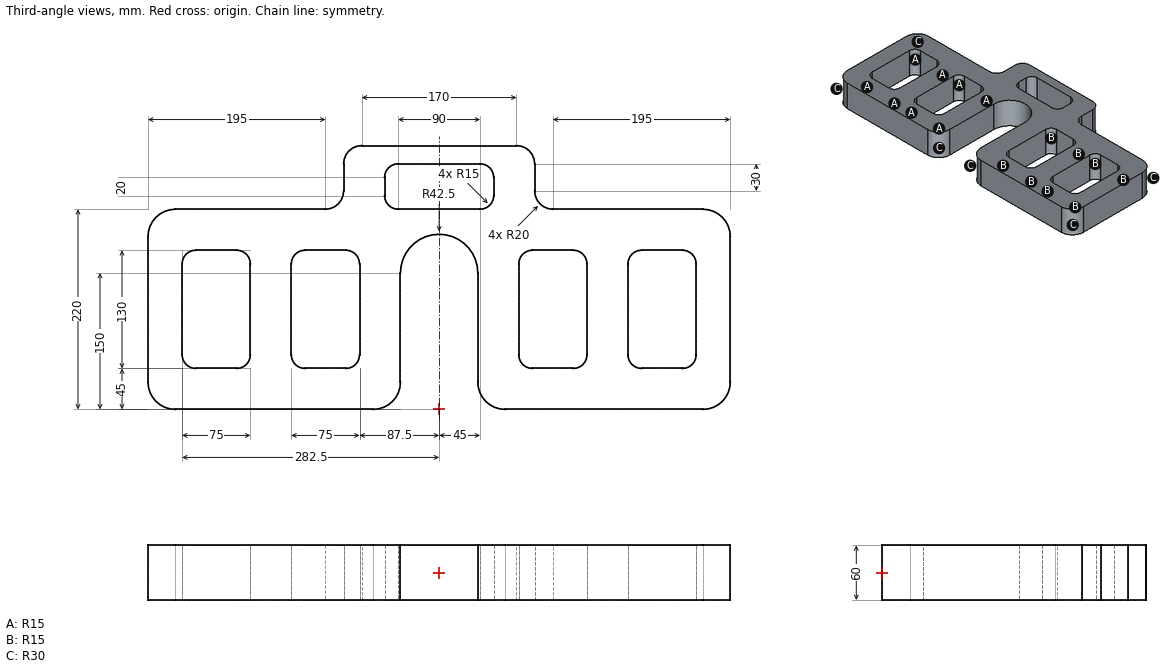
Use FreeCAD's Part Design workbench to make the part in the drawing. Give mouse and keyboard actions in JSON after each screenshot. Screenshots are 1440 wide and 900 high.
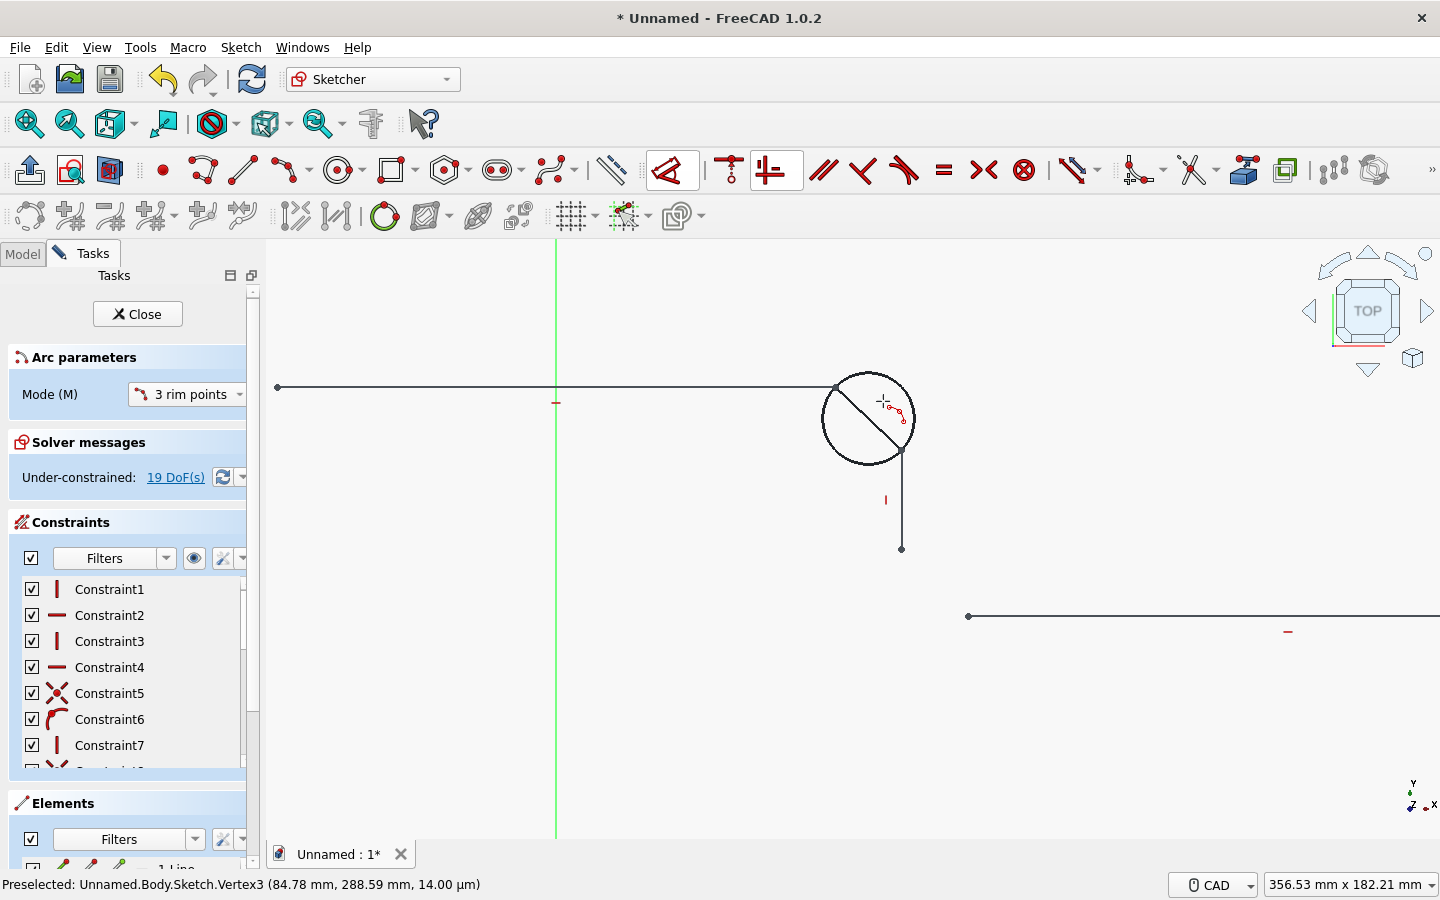
{"action": "left_click", "coordinate": [883, 402]}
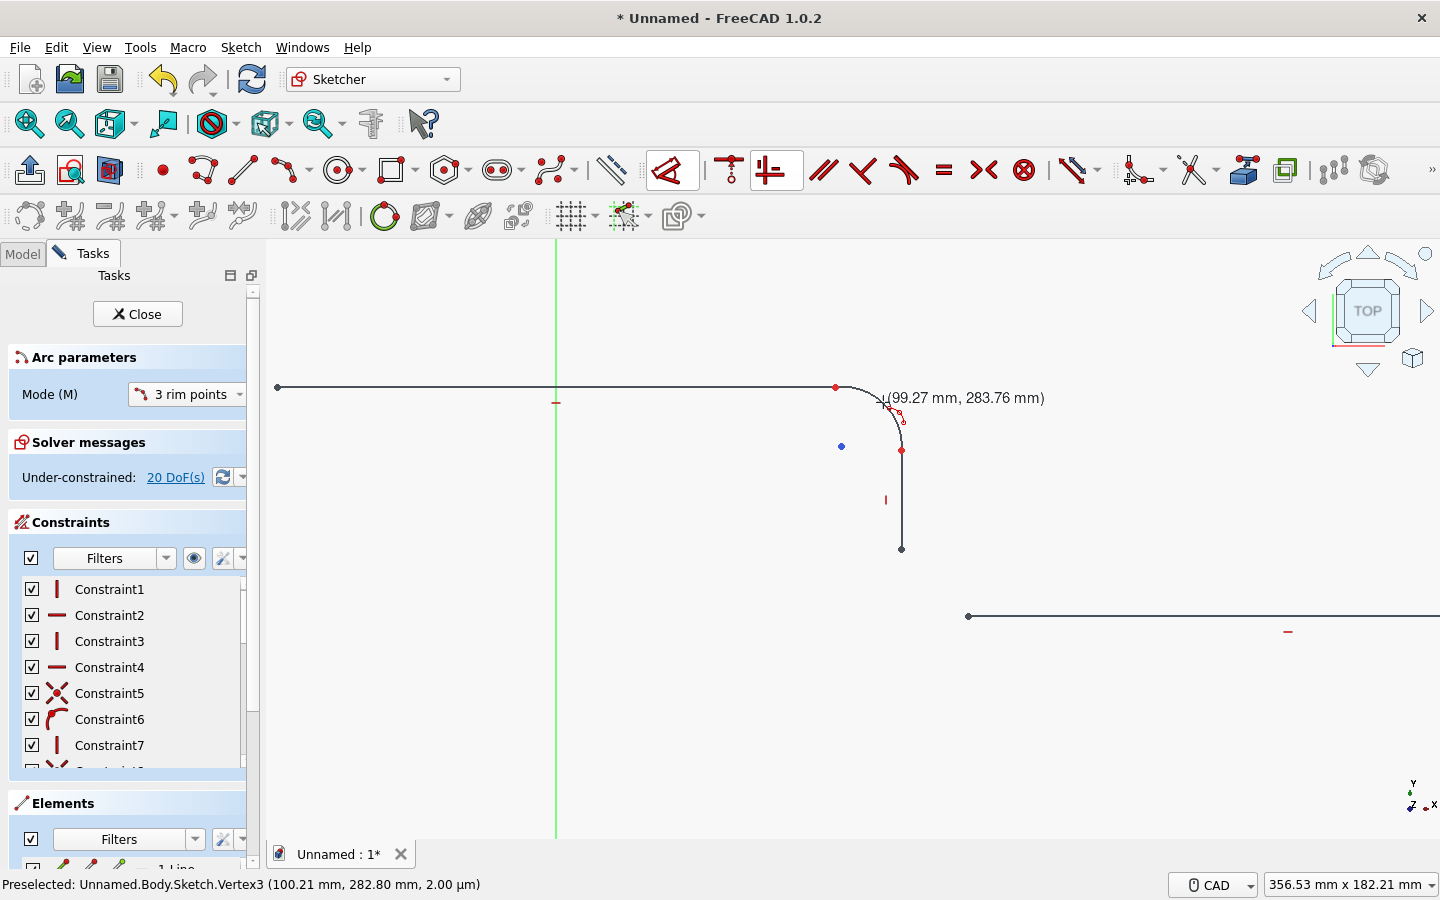
{"action": "scroll", "coordinate": [883, 401], "scroll_direction": "down", "scroll_amount": 6}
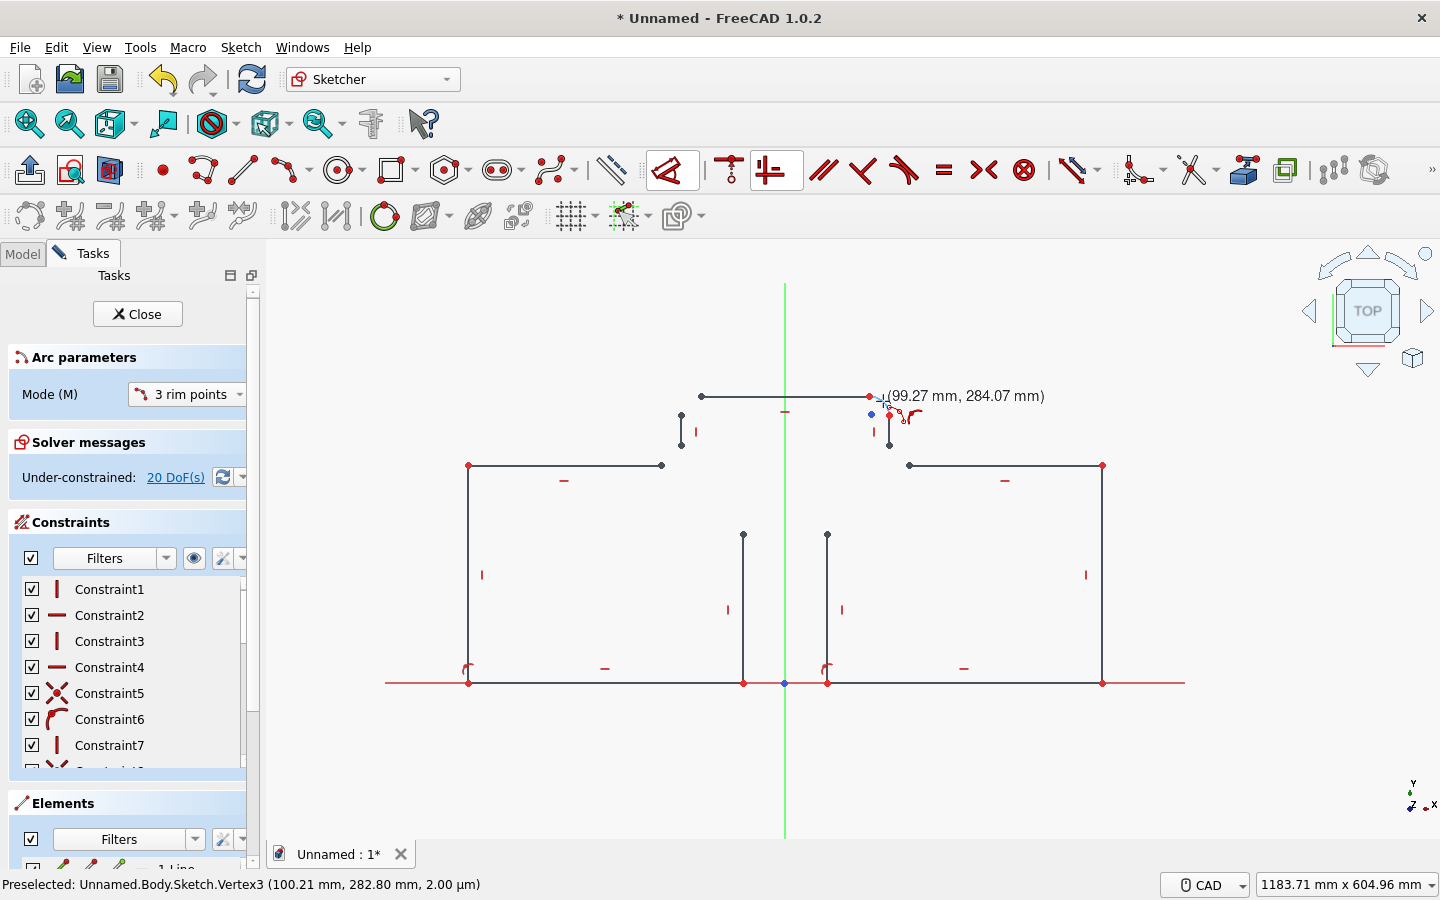
{"action": "left_click", "coordinate": [701, 397]}
{"action": "left_click", "coordinate": [681, 416]}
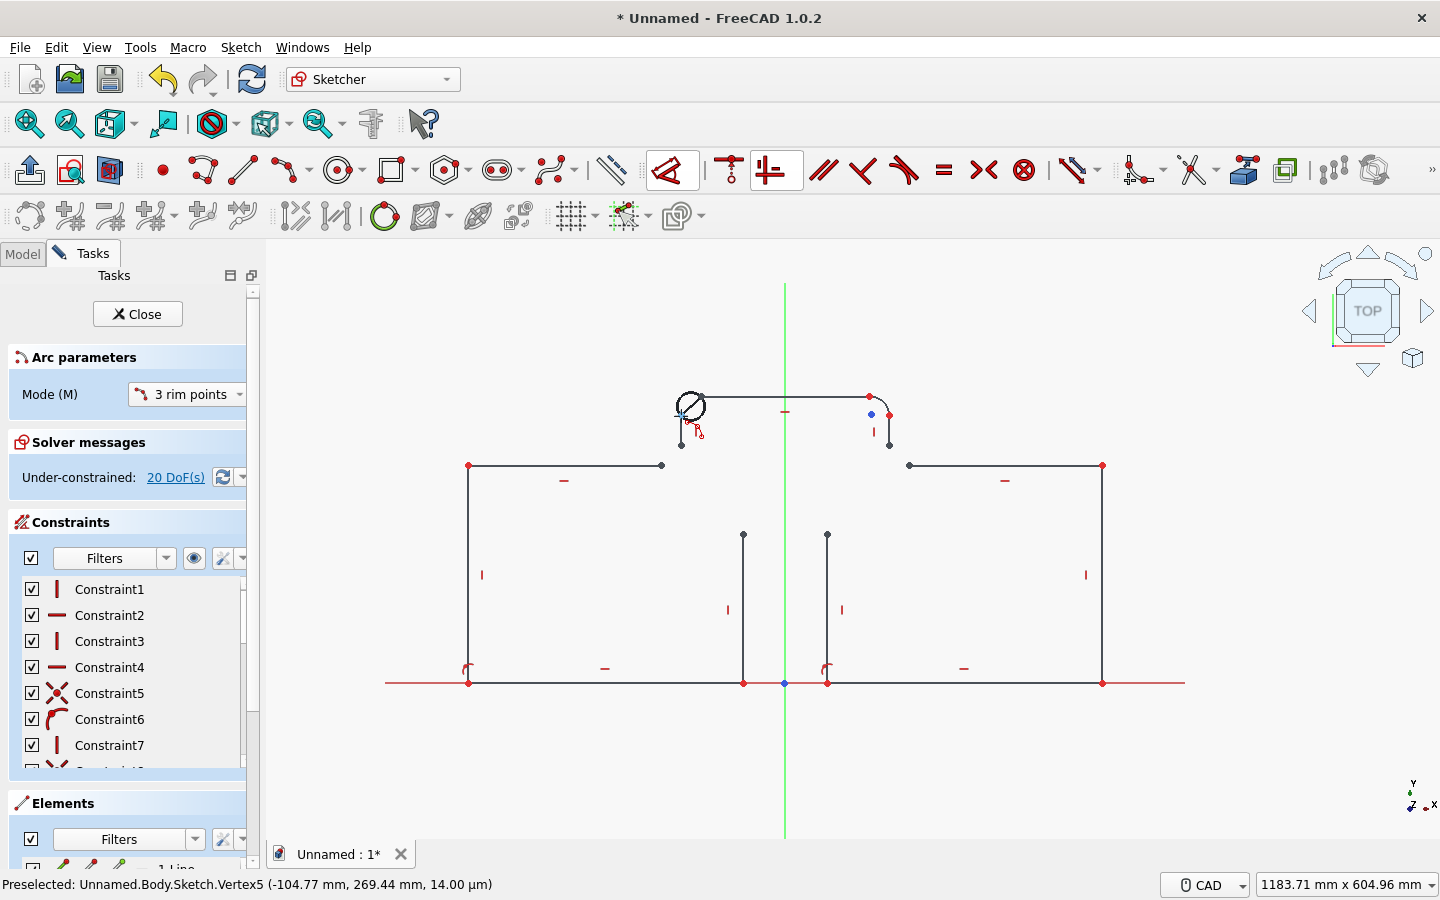
{"action": "scroll", "coordinate": [687, 401], "scroll_direction": "up", "scroll_amount": 6}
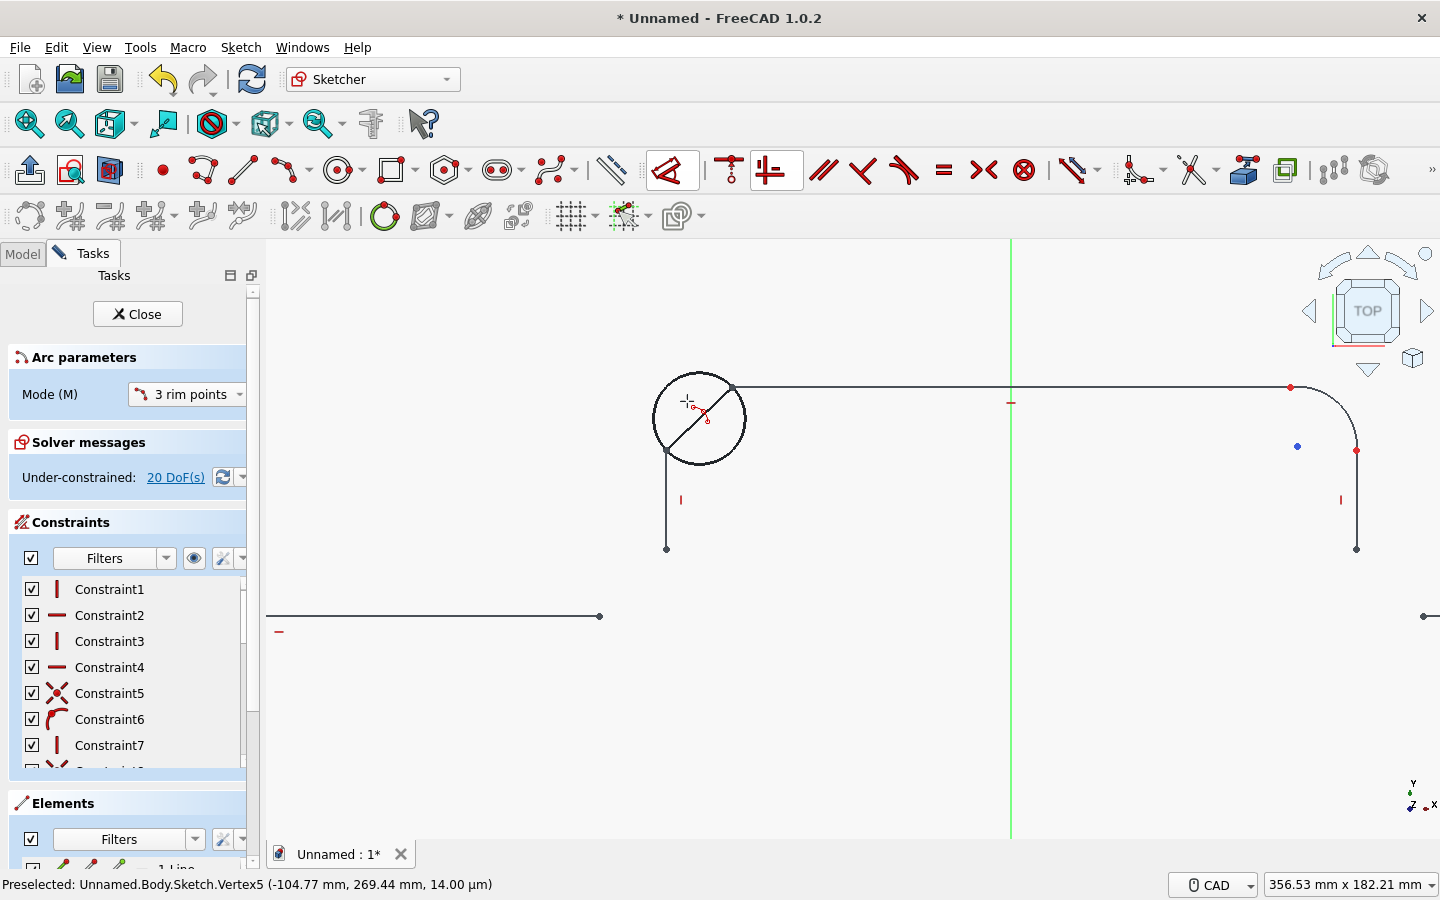
{"action": "left_click", "coordinate": [685, 402]}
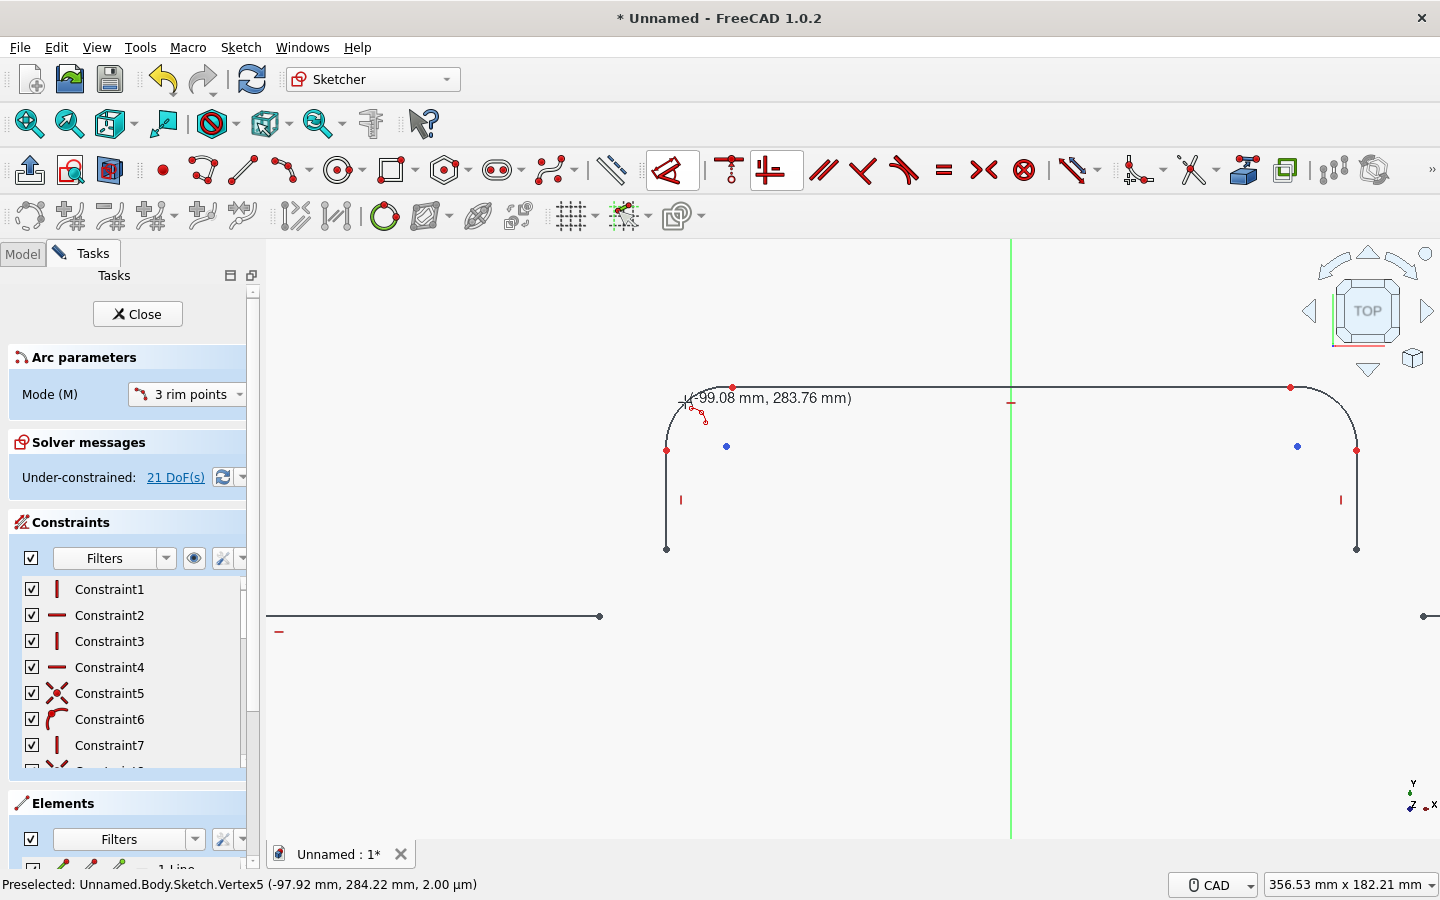
{"action": "left_click", "coordinate": [666, 550]}
{"action": "left_click", "coordinate": [600, 616]}
{"action": "left_click", "coordinate": [646, 594]}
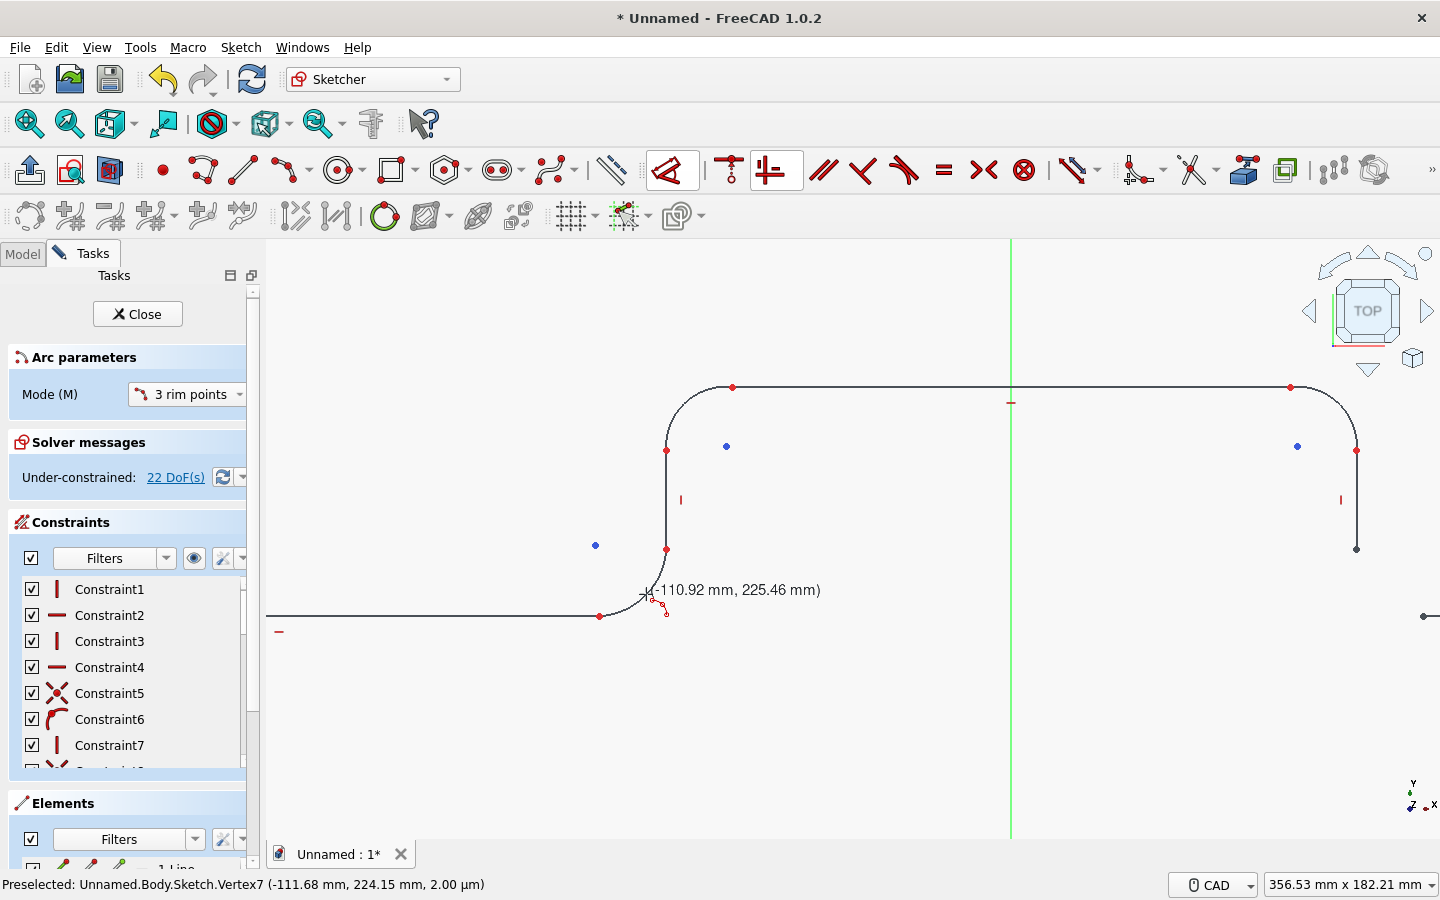
{"action": "scroll", "coordinate": [687, 401], "scroll_direction": "down", "scroll_amount": 6}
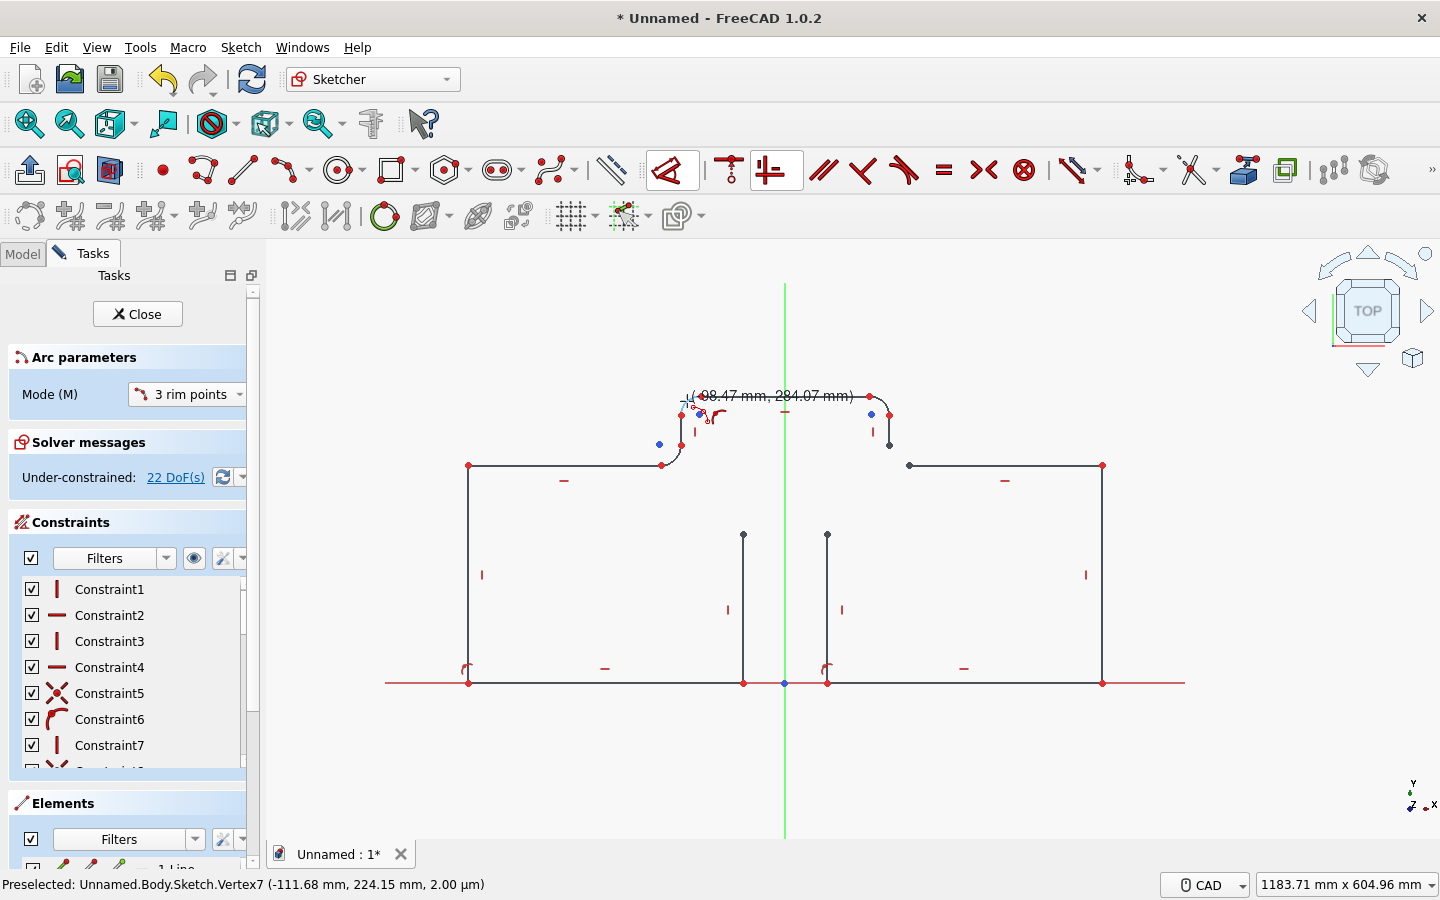
{"action": "left_click", "coordinate": [743, 535]}
{"action": "left_click", "coordinate": [827, 535]}
{"action": "left_click", "coordinate": [810, 500]}